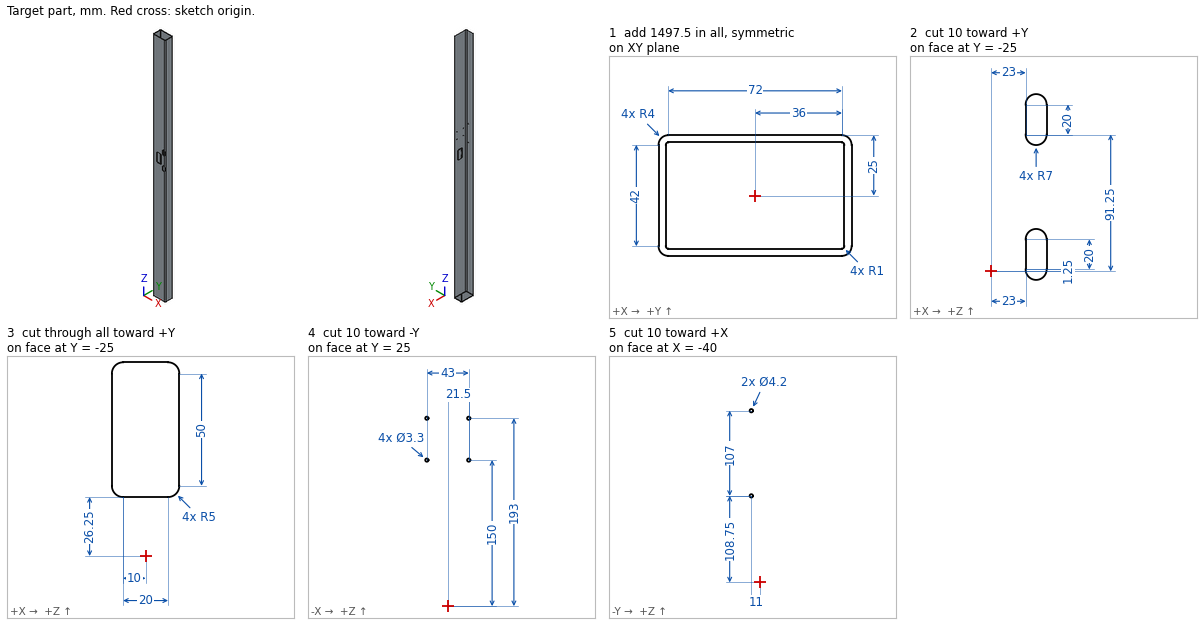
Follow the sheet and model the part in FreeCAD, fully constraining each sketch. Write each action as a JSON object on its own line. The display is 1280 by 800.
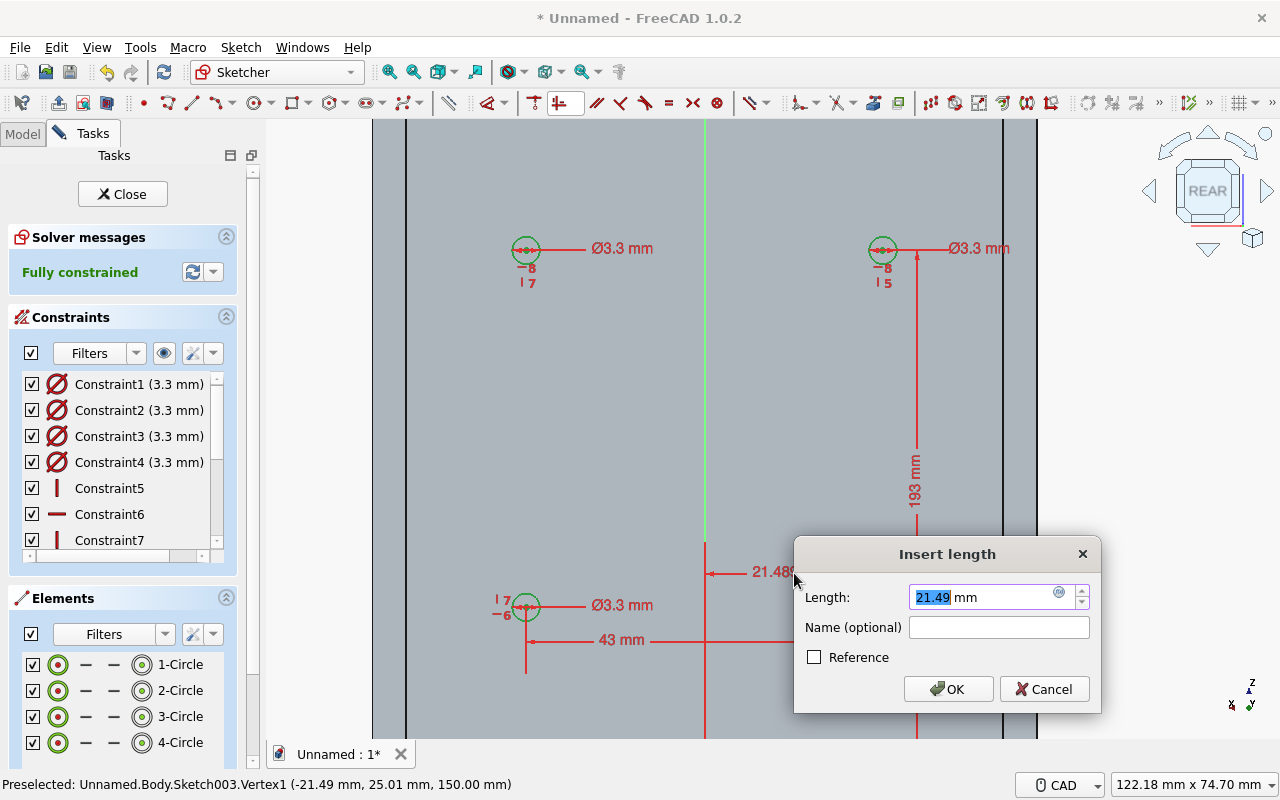
{"action": "type", "text": "21.5"}
{"action": "key", "text": "Return"}
{"action": "key", "text": "Escape"}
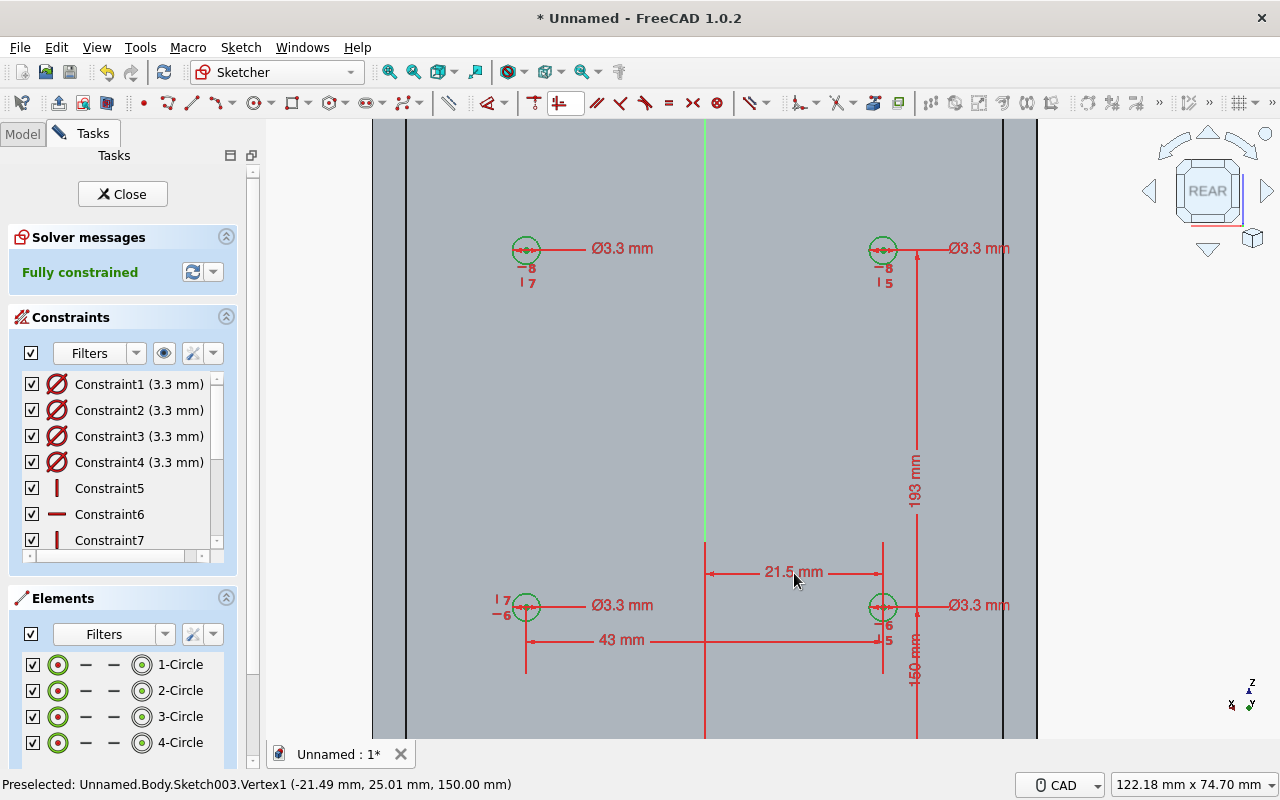
{"action": "left_click", "coordinate": [123, 194]}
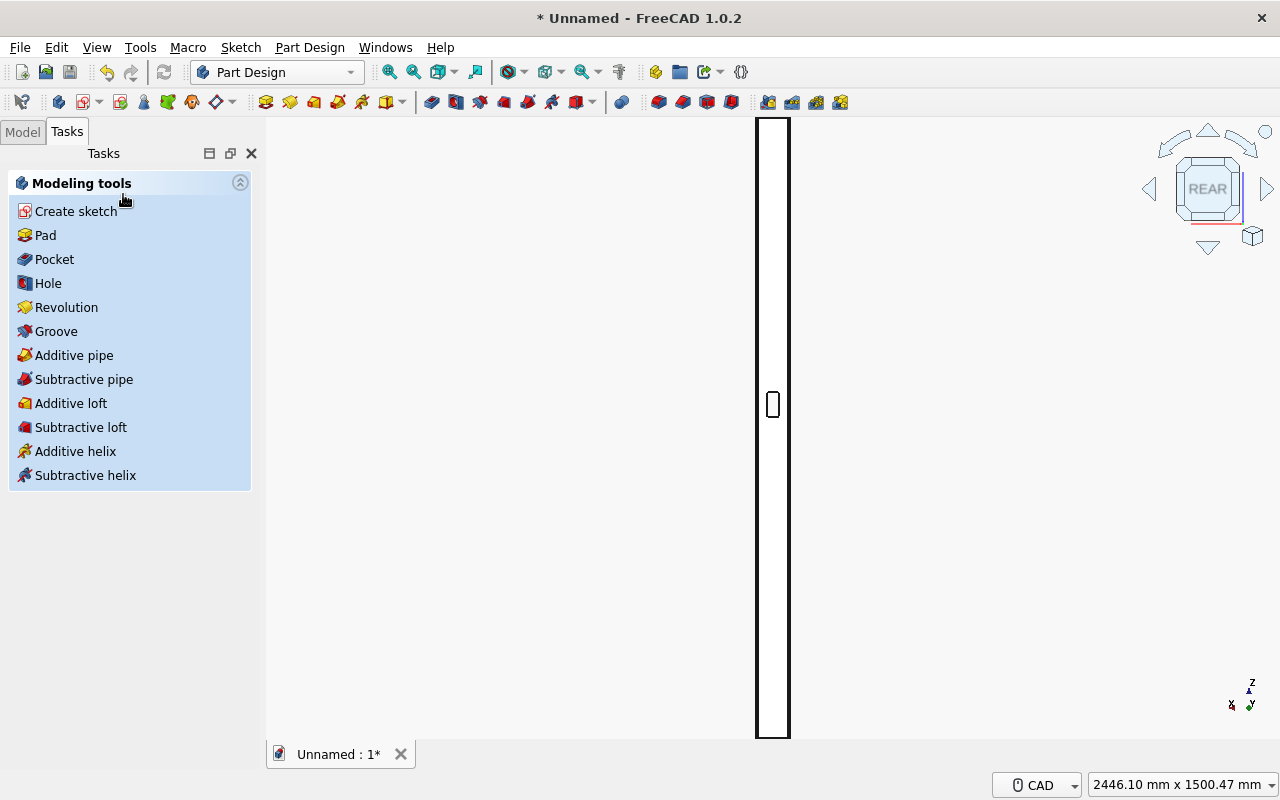
{"action": "left_click", "coordinate": [432, 102]}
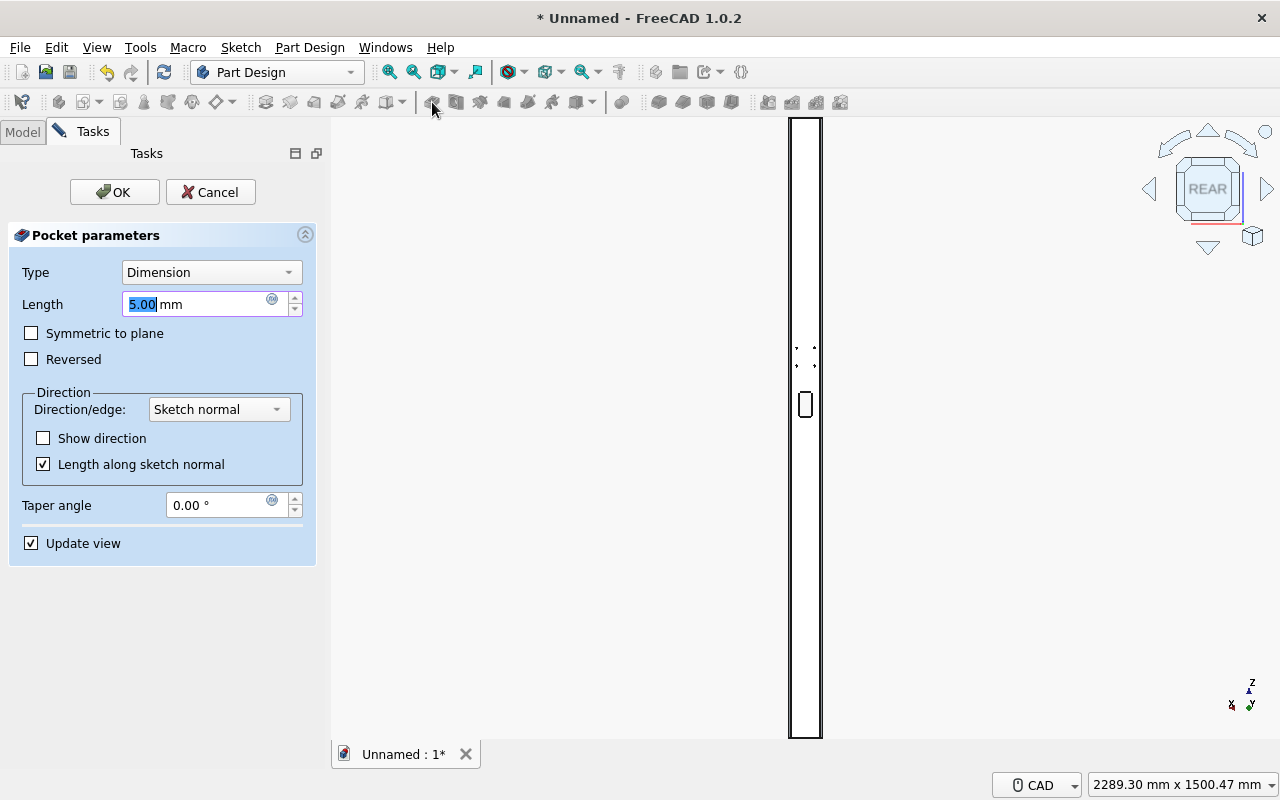
{"action": "type", "text": "10"}
{"action": "key", "text": "Tab"}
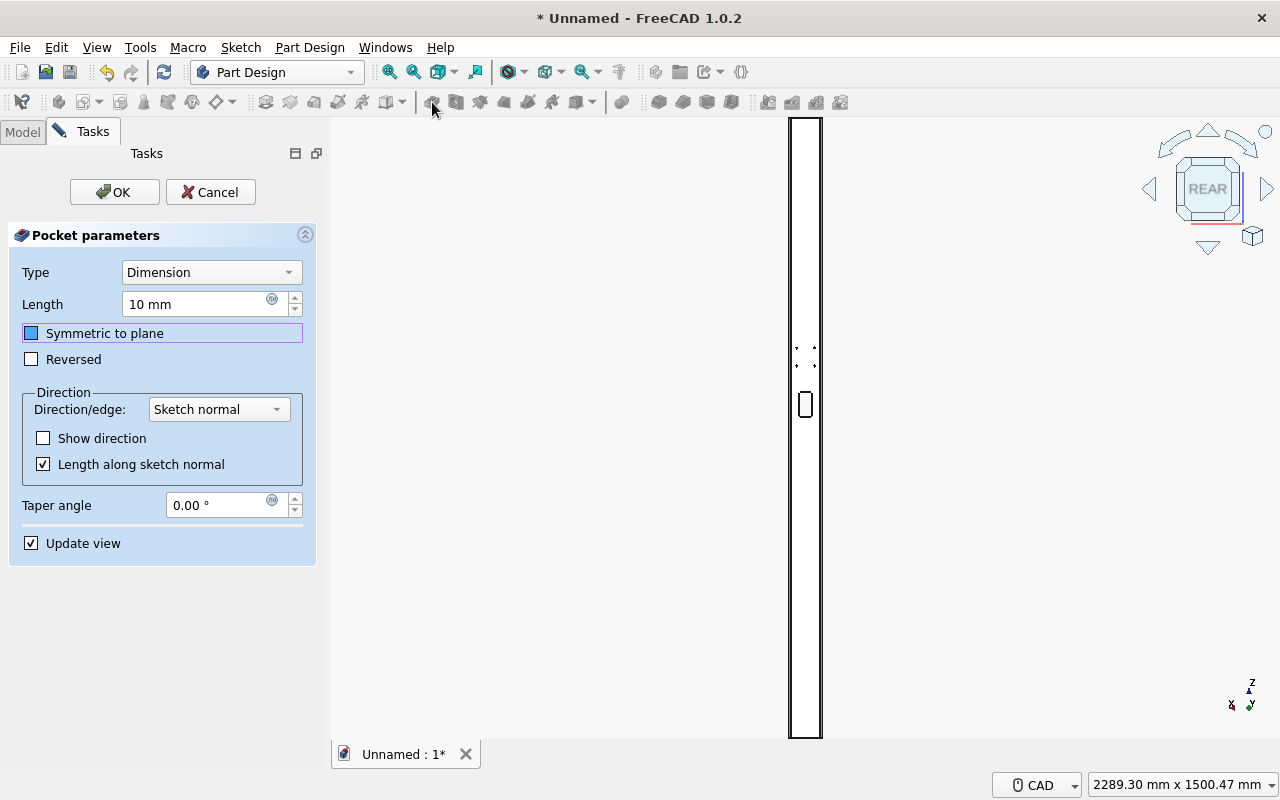
{"action": "left_click", "coordinate": [115, 192]}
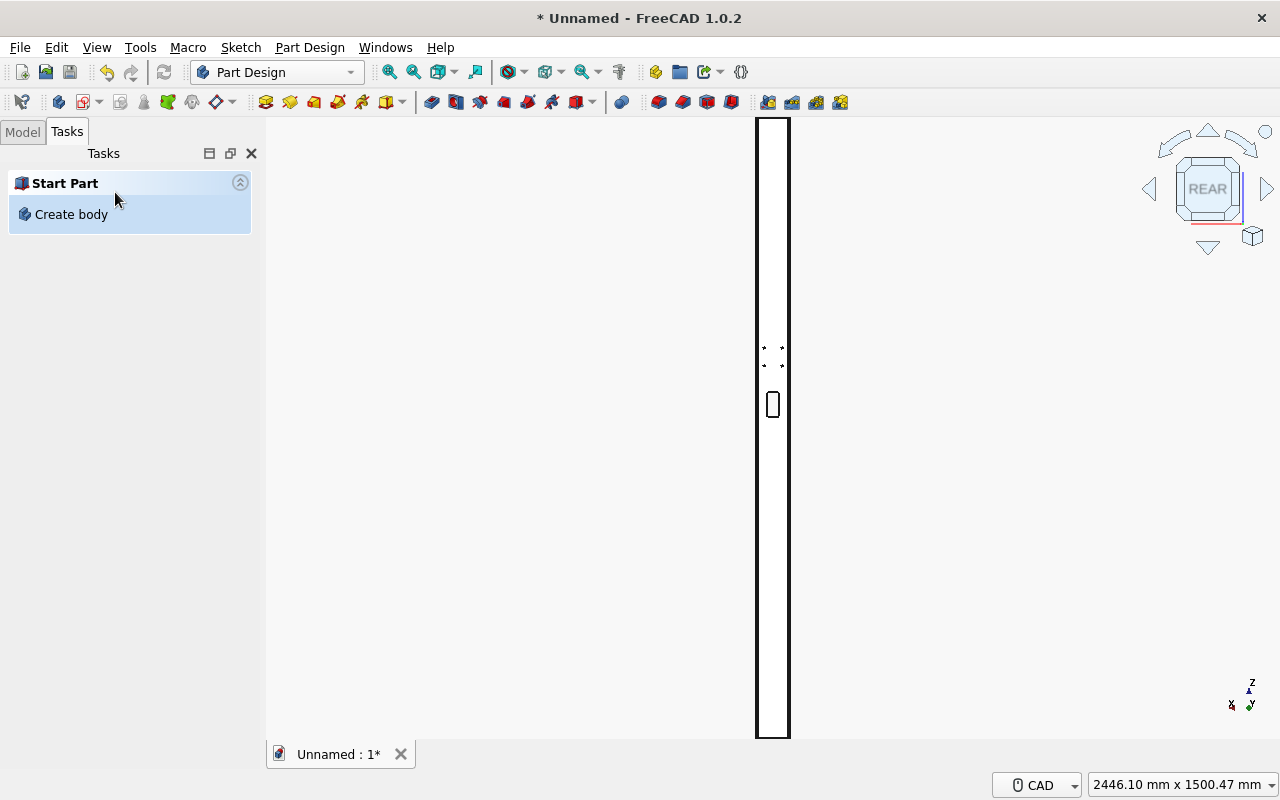
{"action": "key", "text": "6"}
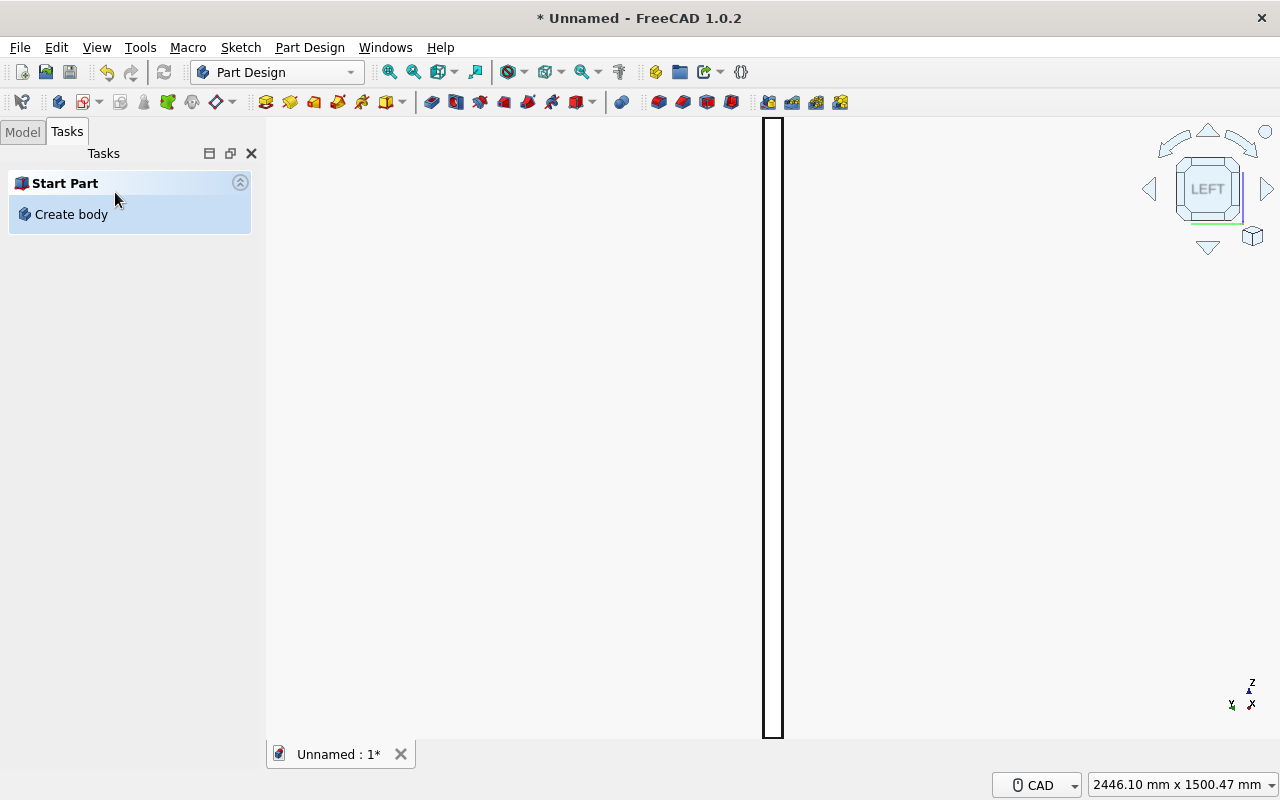
{"action": "left_click", "coordinate": [773, 161]}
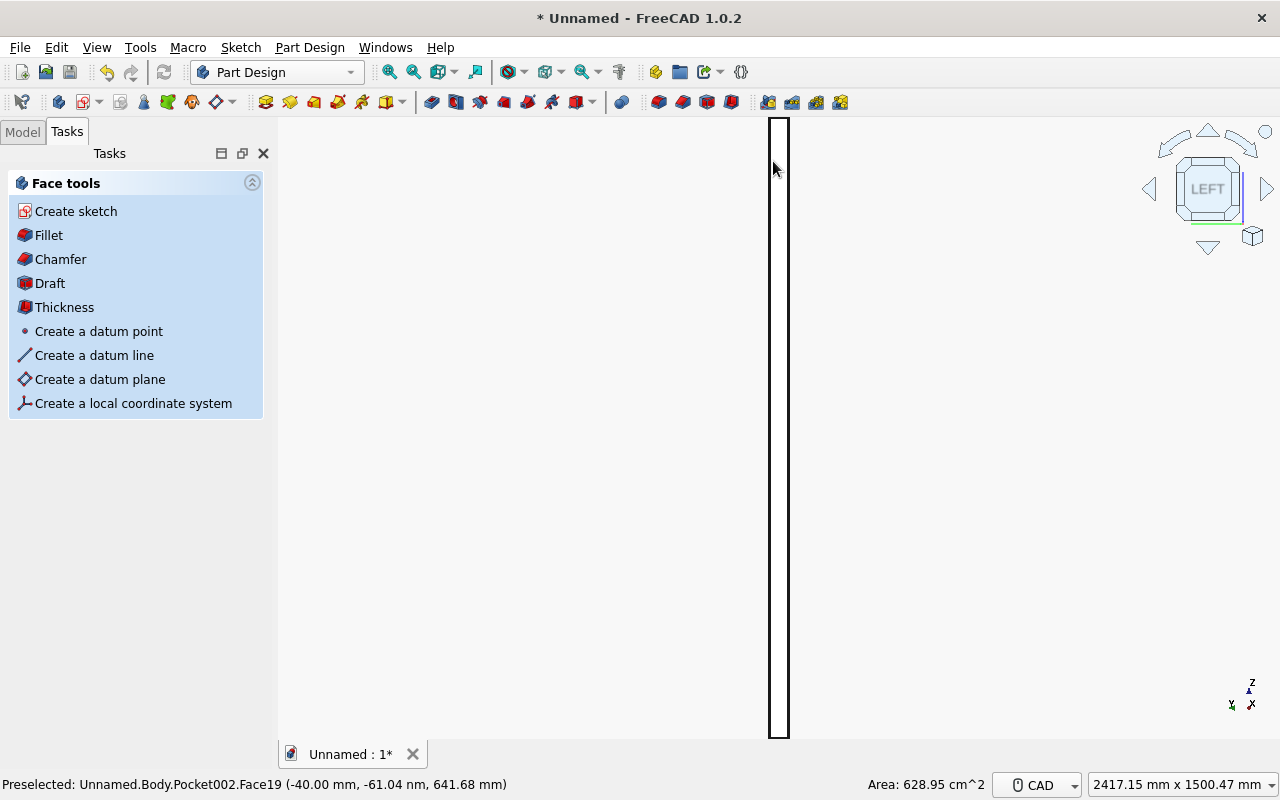
{"action": "left_click", "coordinate": [84, 102]}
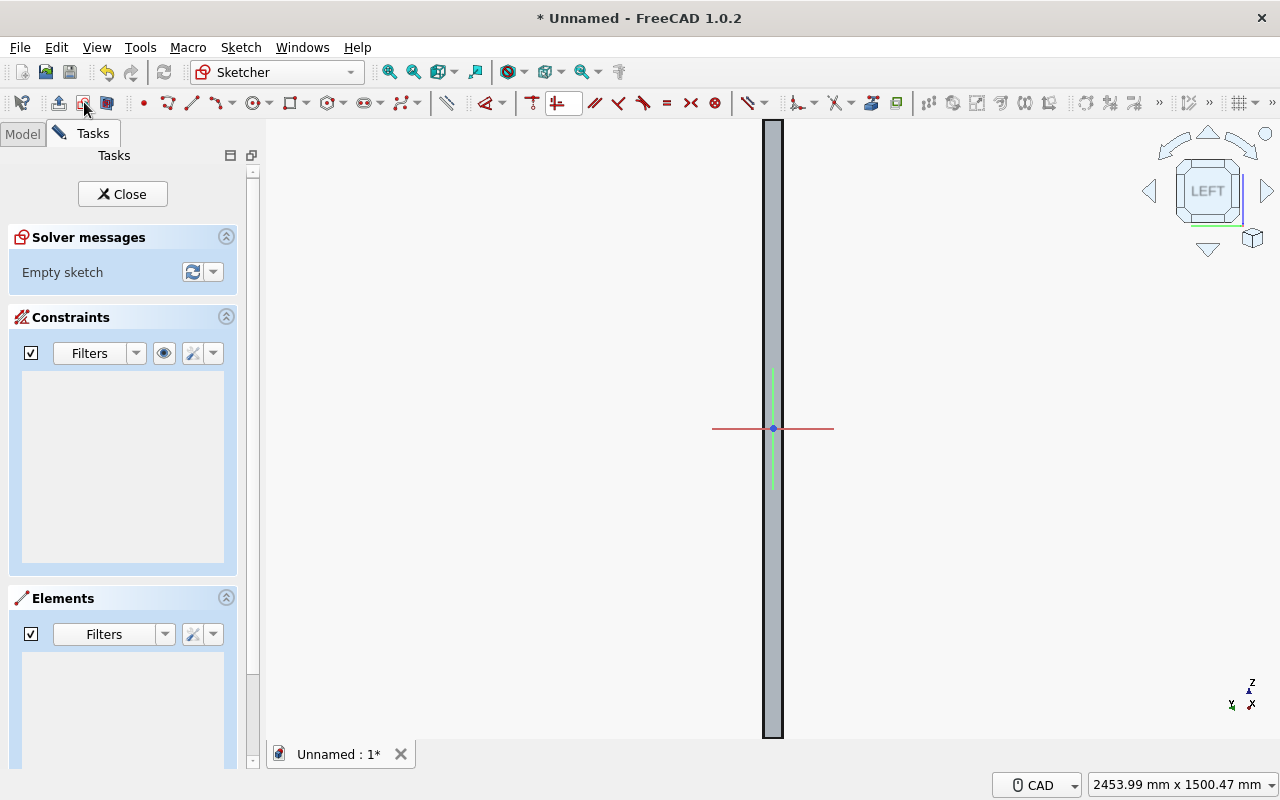
{"action": "scroll", "coordinate": [792, 369], "scroll_direction": "up", "scroll_amount": 7}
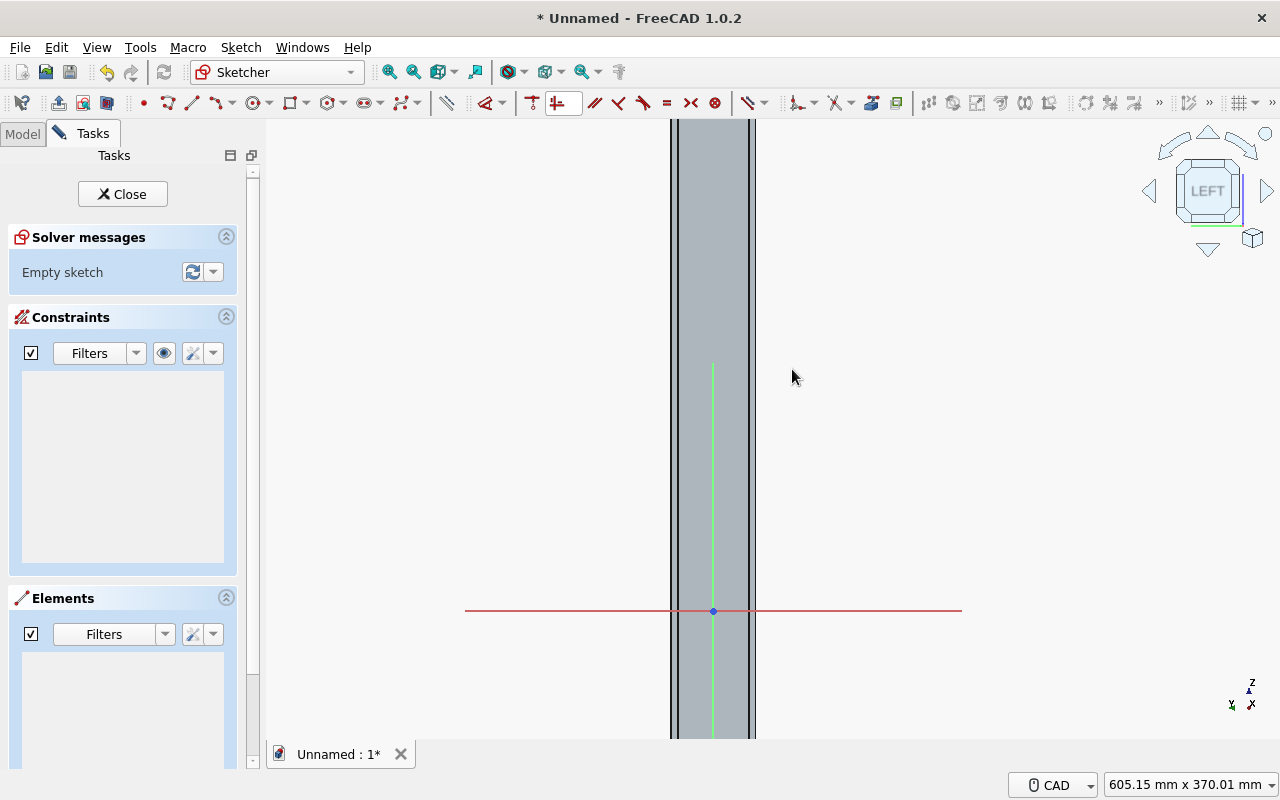
{"action": "left_click", "coordinate": [254, 104]}